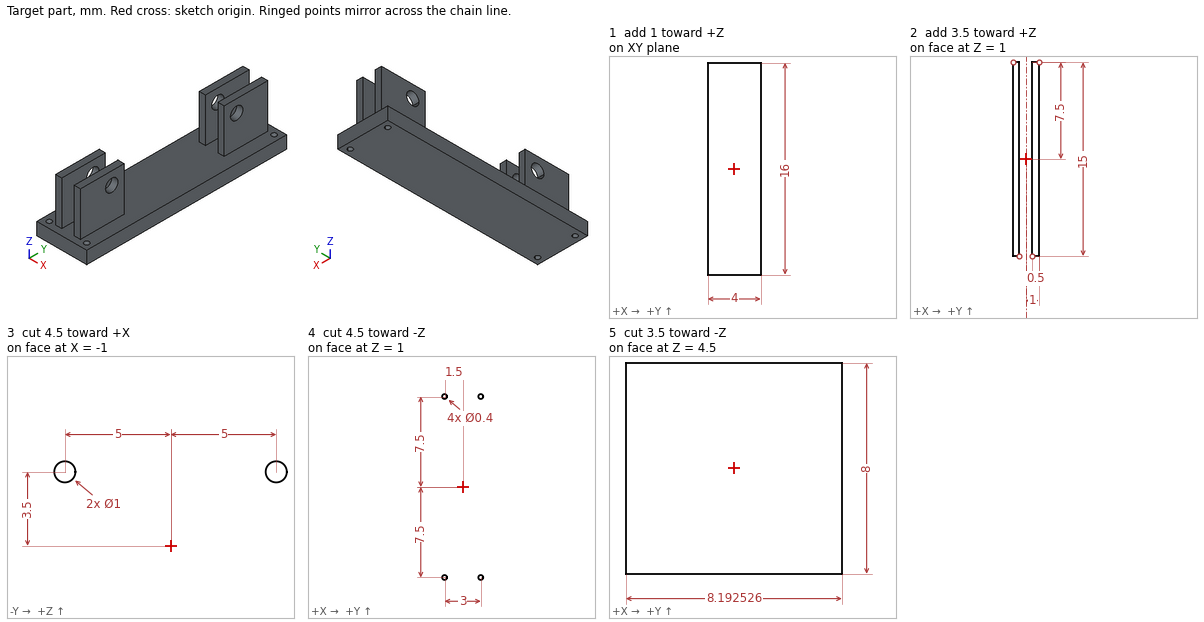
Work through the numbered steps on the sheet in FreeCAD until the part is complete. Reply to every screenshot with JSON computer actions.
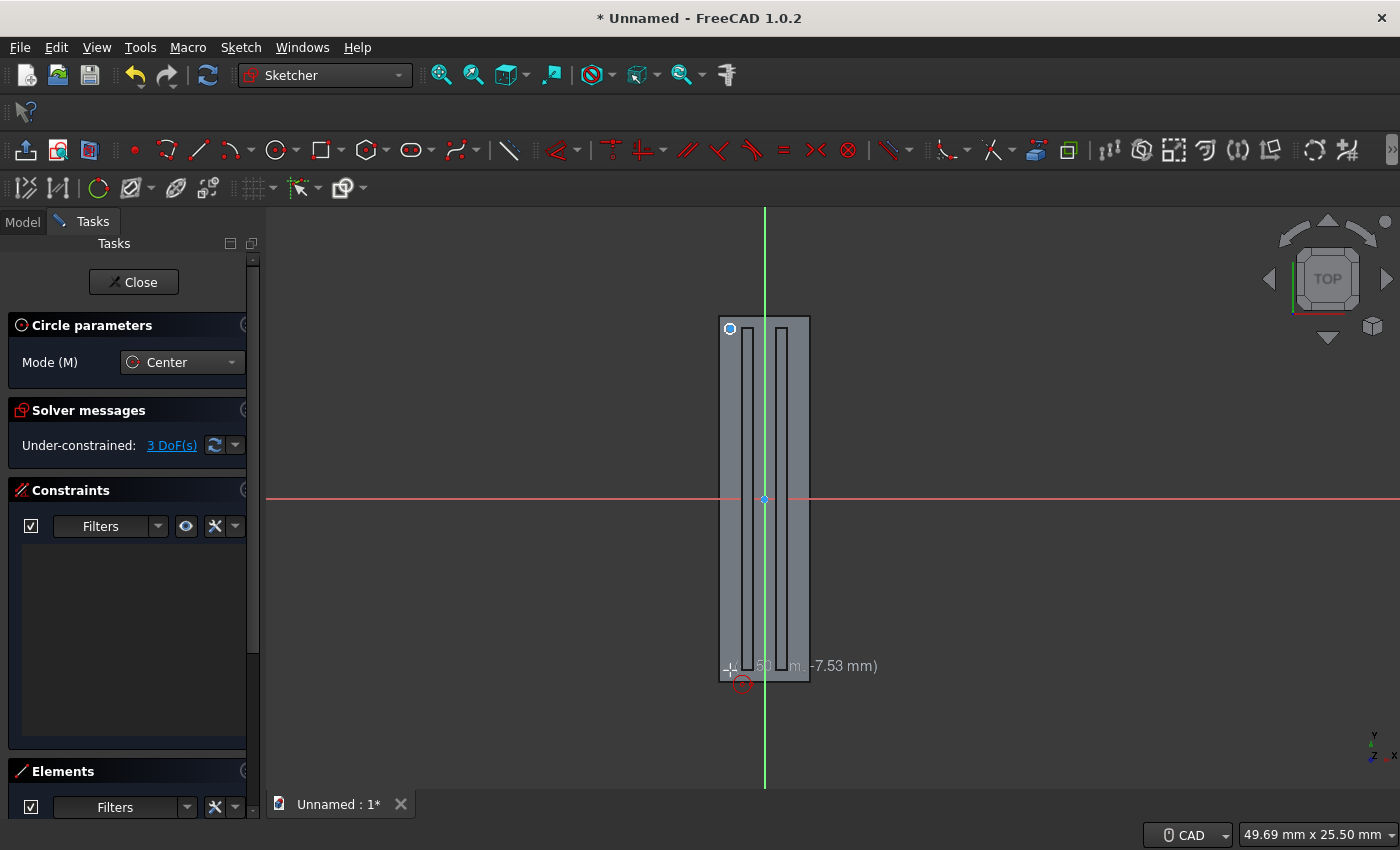
{"action": "left_click", "coordinate": [730, 670]}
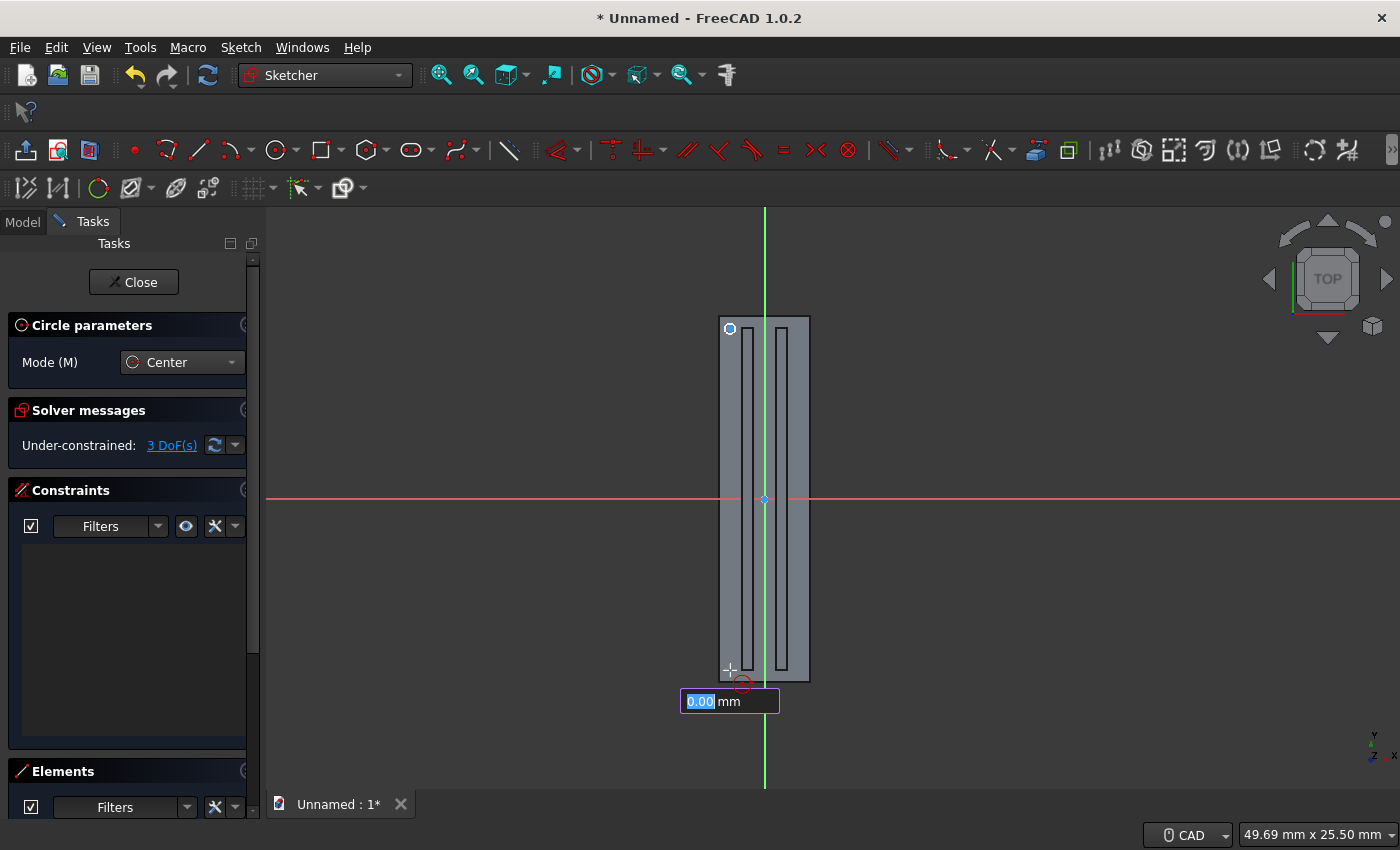
{"action": "scroll", "coordinate": [734, 667], "scroll_direction": "up", "scroll_amount": 7}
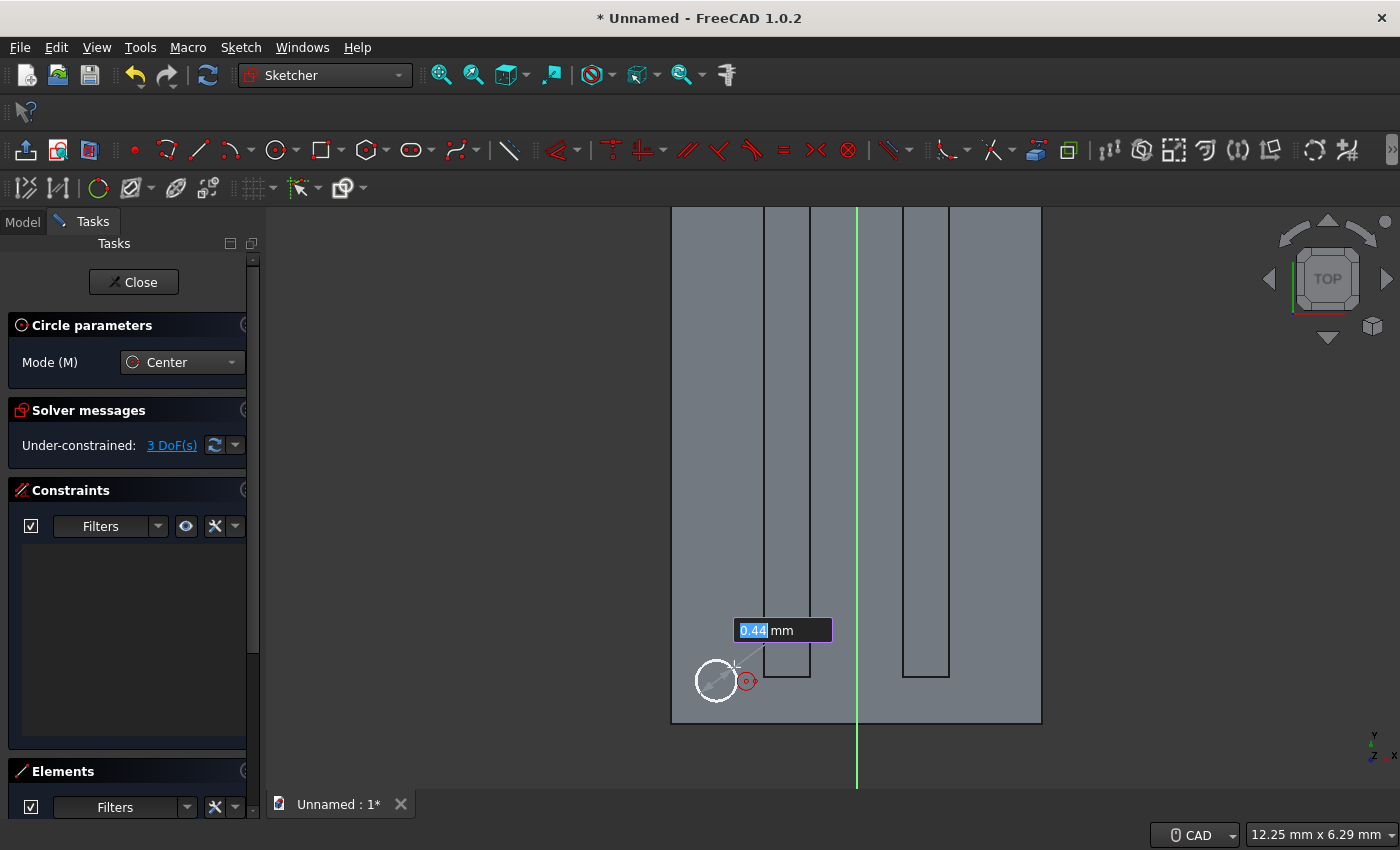
{"action": "left_click", "coordinate": [731, 664]}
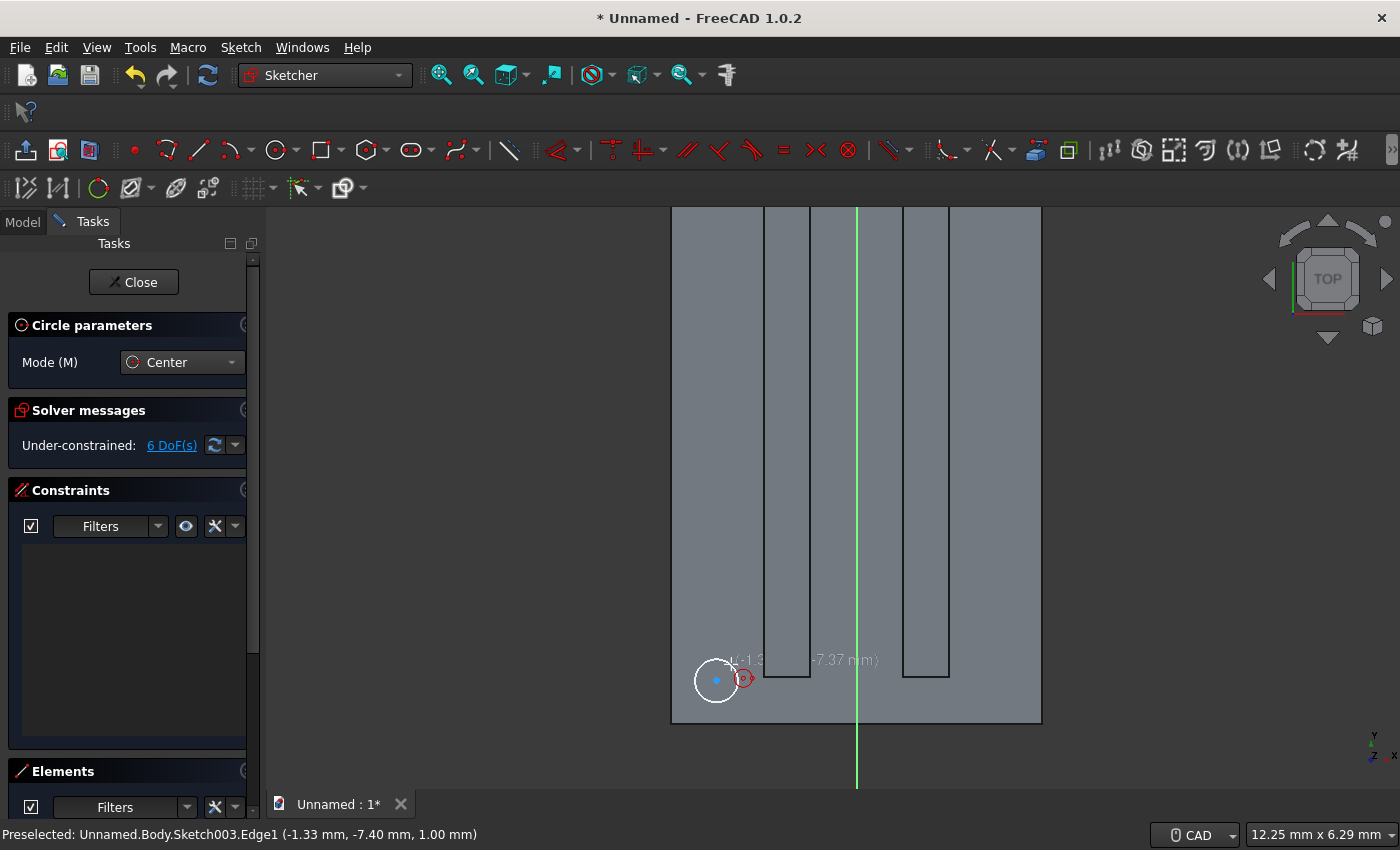
{"action": "scroll", "coordinate": [995, 677], "scroll_direction": "up", "scroll_amount": 2}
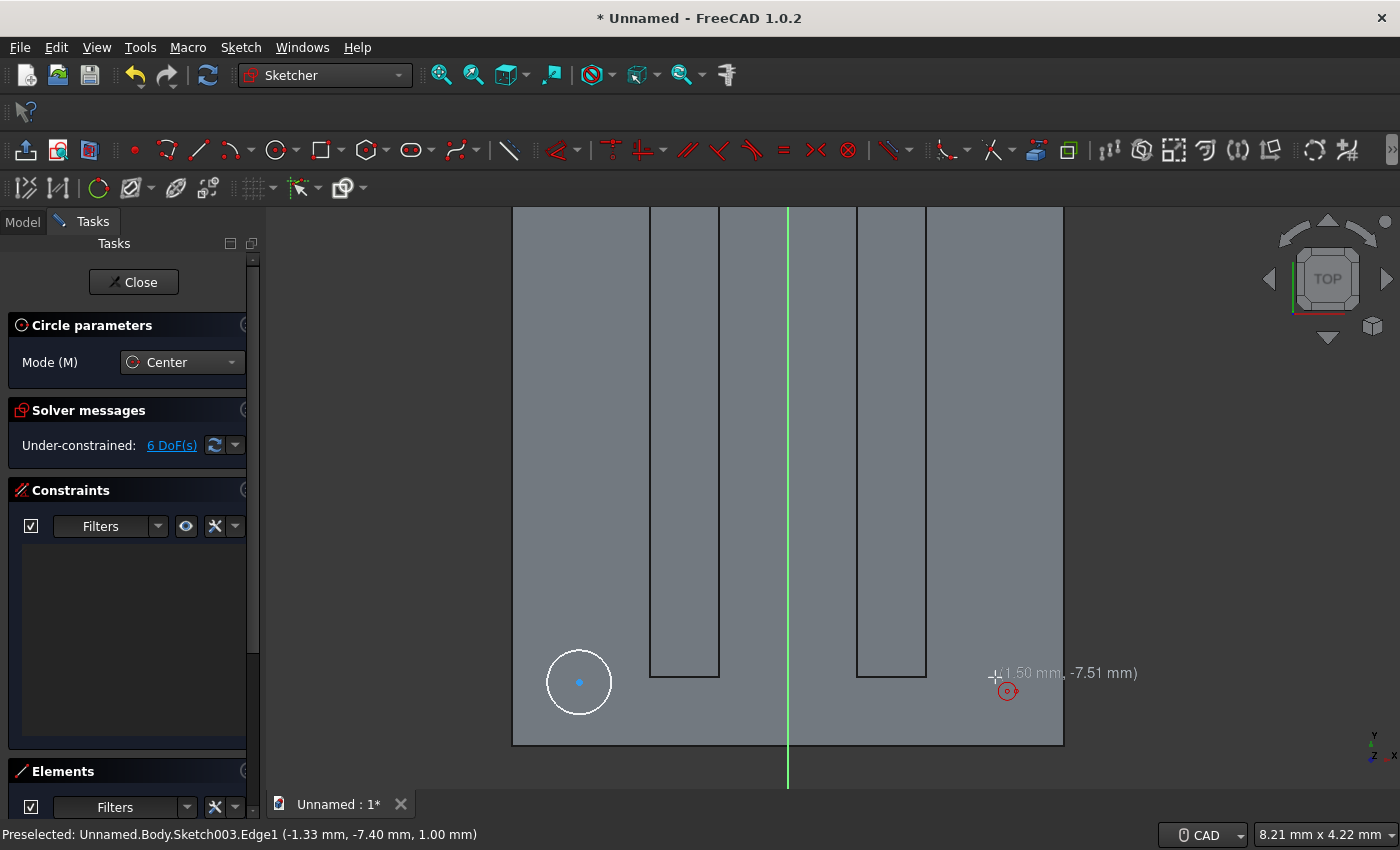
{"action": "scroll", "coordinate": [760, 668], "scroll_direction": "down", "scroll_amount": 9}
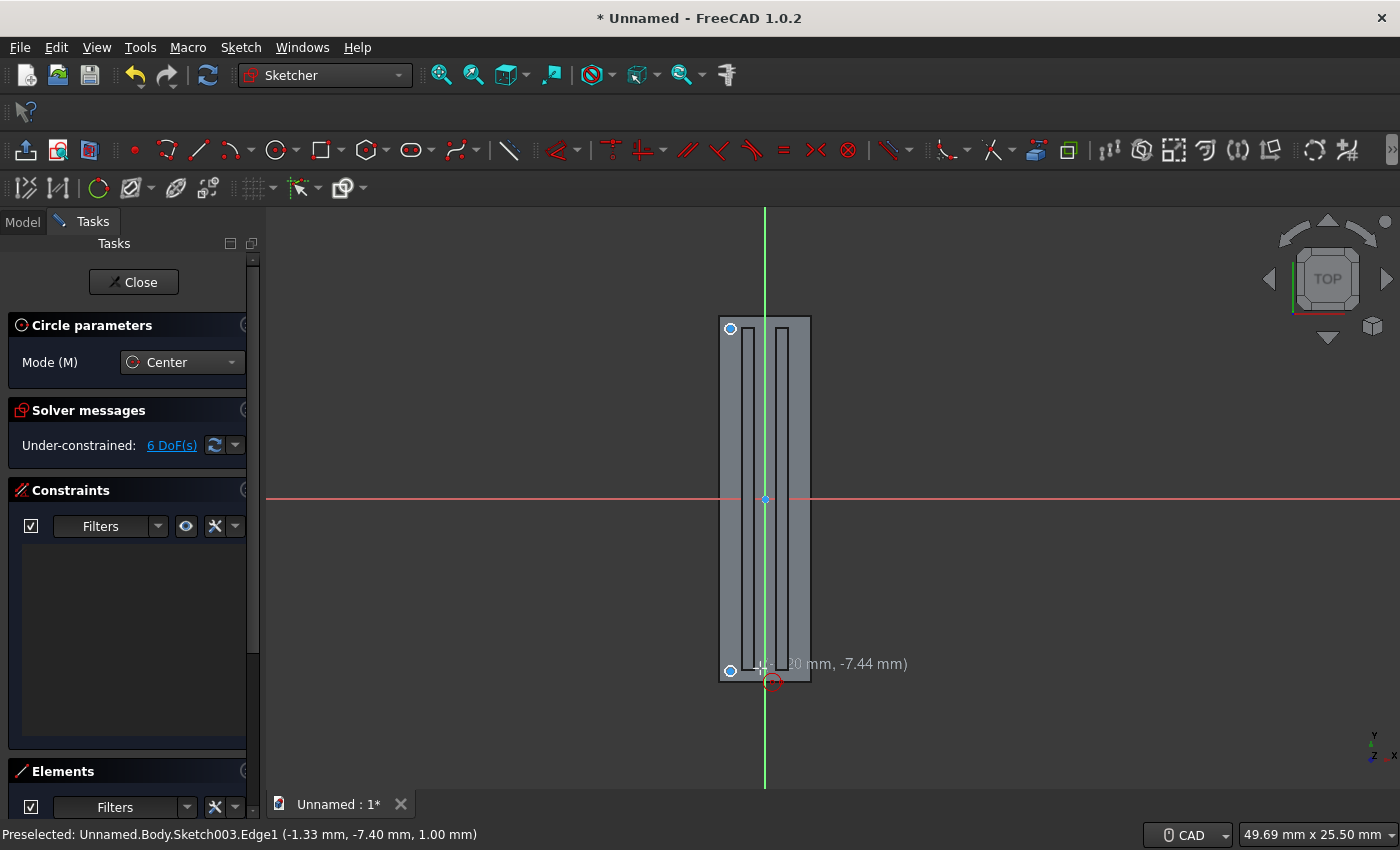
{"action": "left_click", "coordinate": [799, 670]}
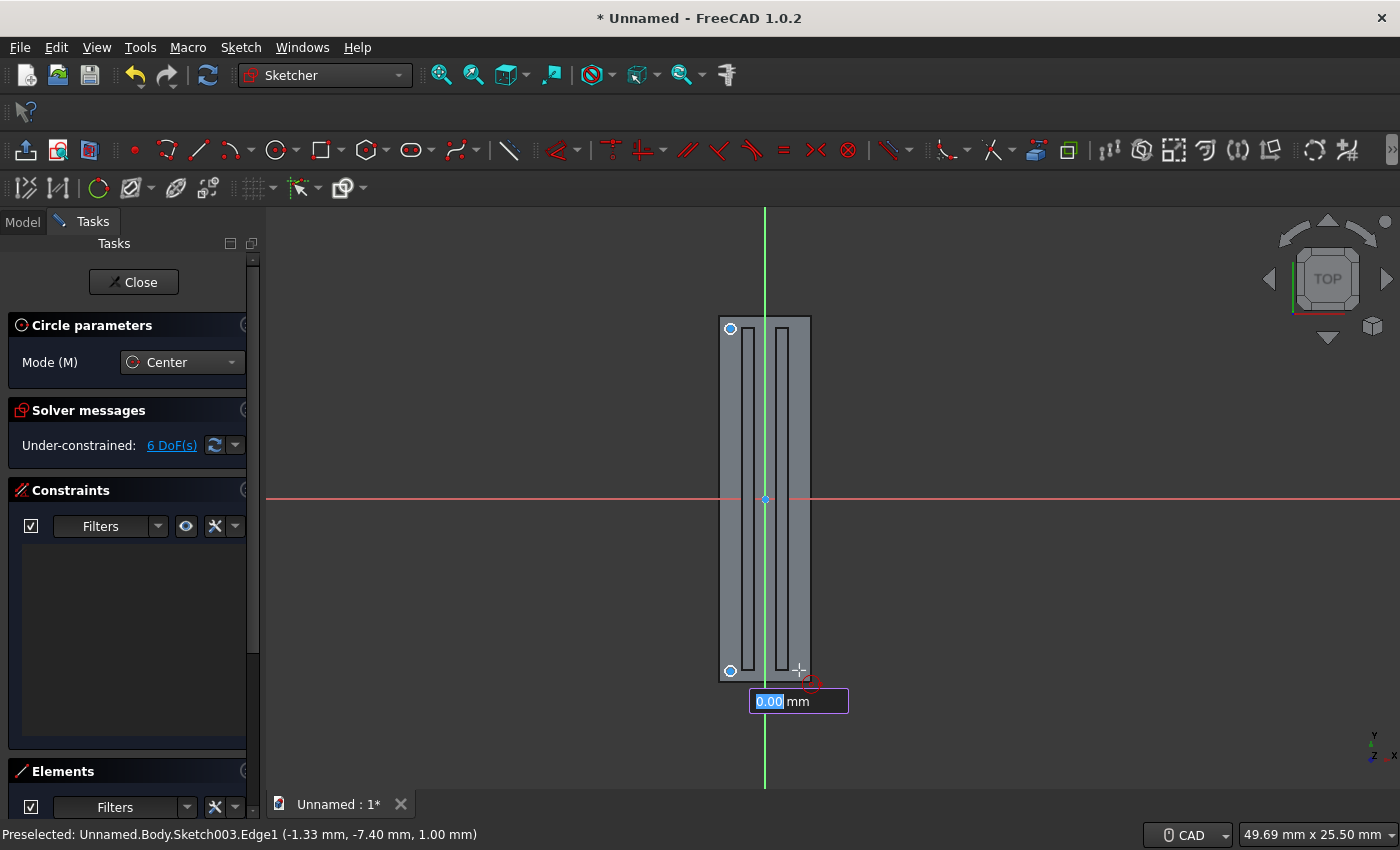
{"action": "scroll", "coordinate": [802, 667], "scroll_direction": "up", "scroll_amount": 7}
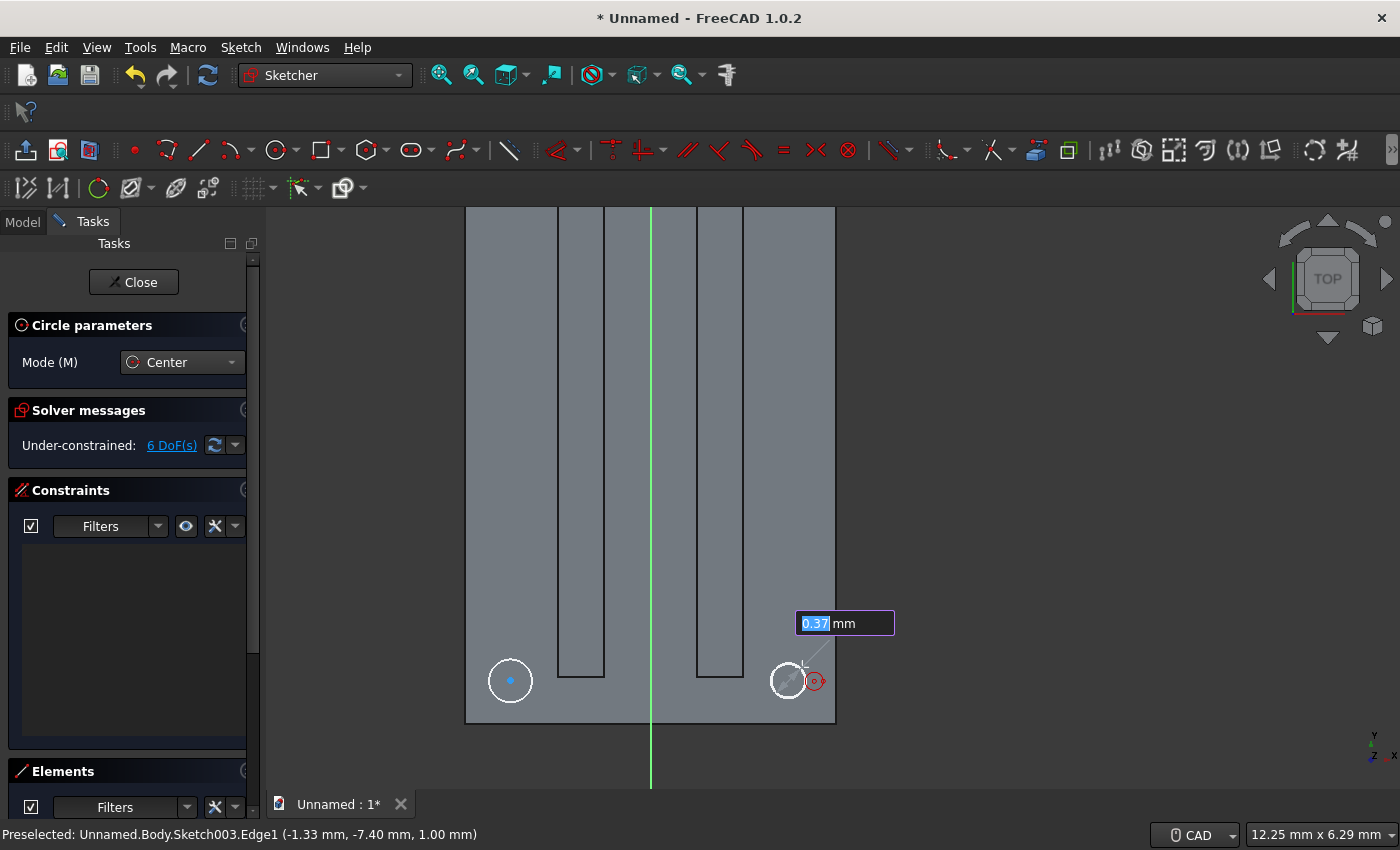
{"action": "left_click", "coordinate": [802, 664]}